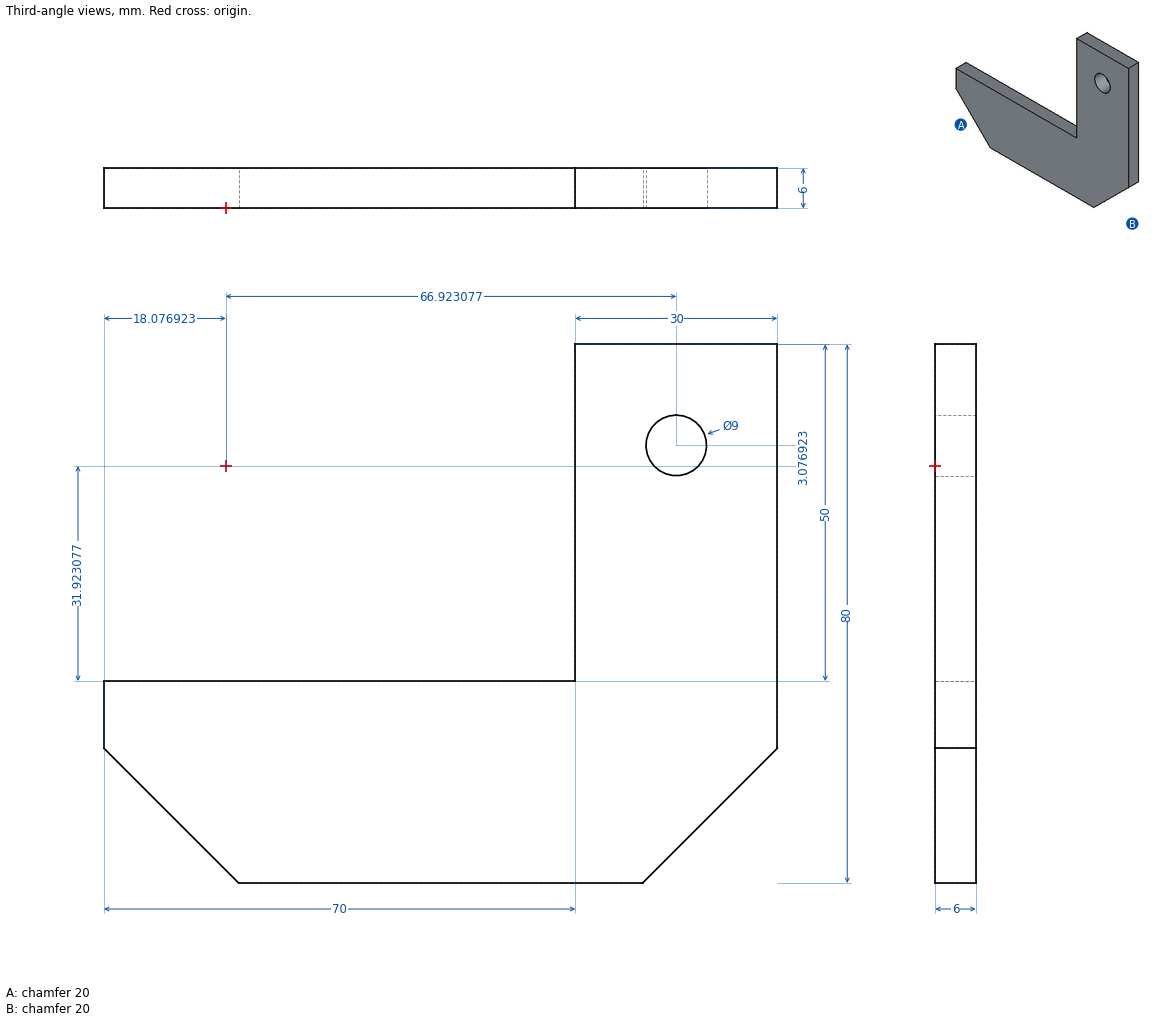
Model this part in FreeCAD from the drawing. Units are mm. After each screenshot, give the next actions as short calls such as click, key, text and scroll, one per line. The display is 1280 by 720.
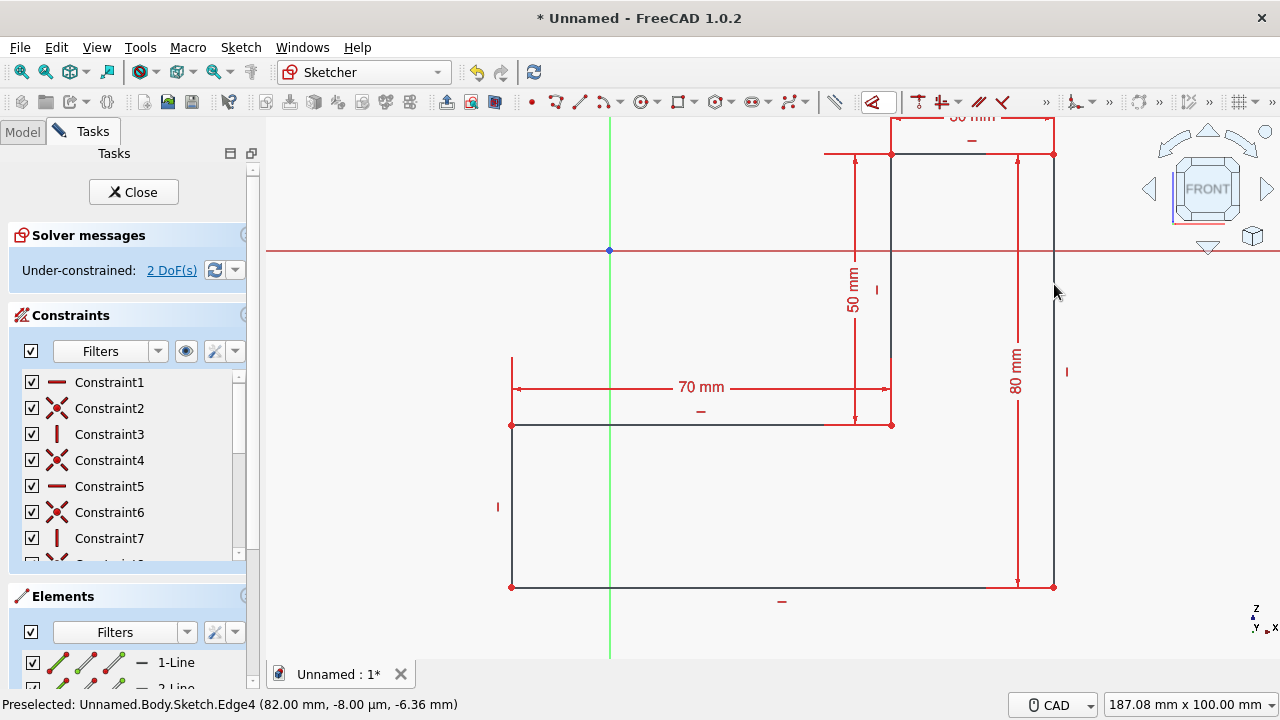
click(512, 425)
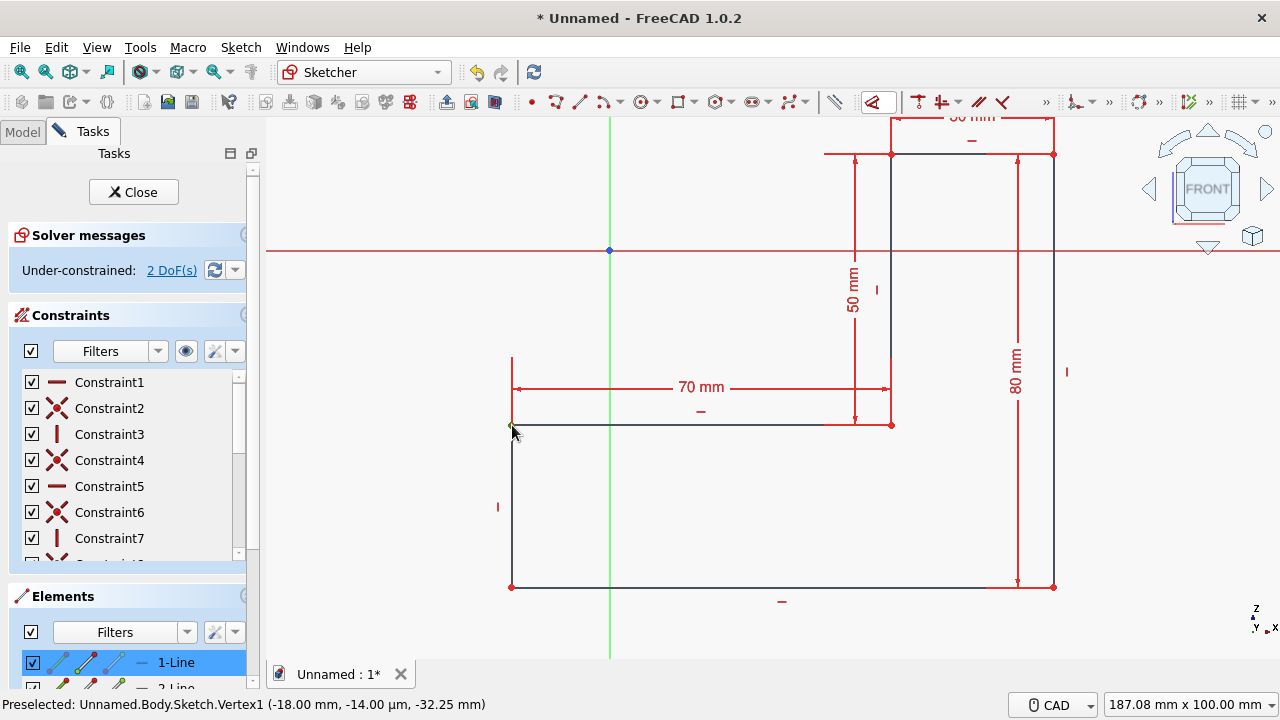
click(890, 102)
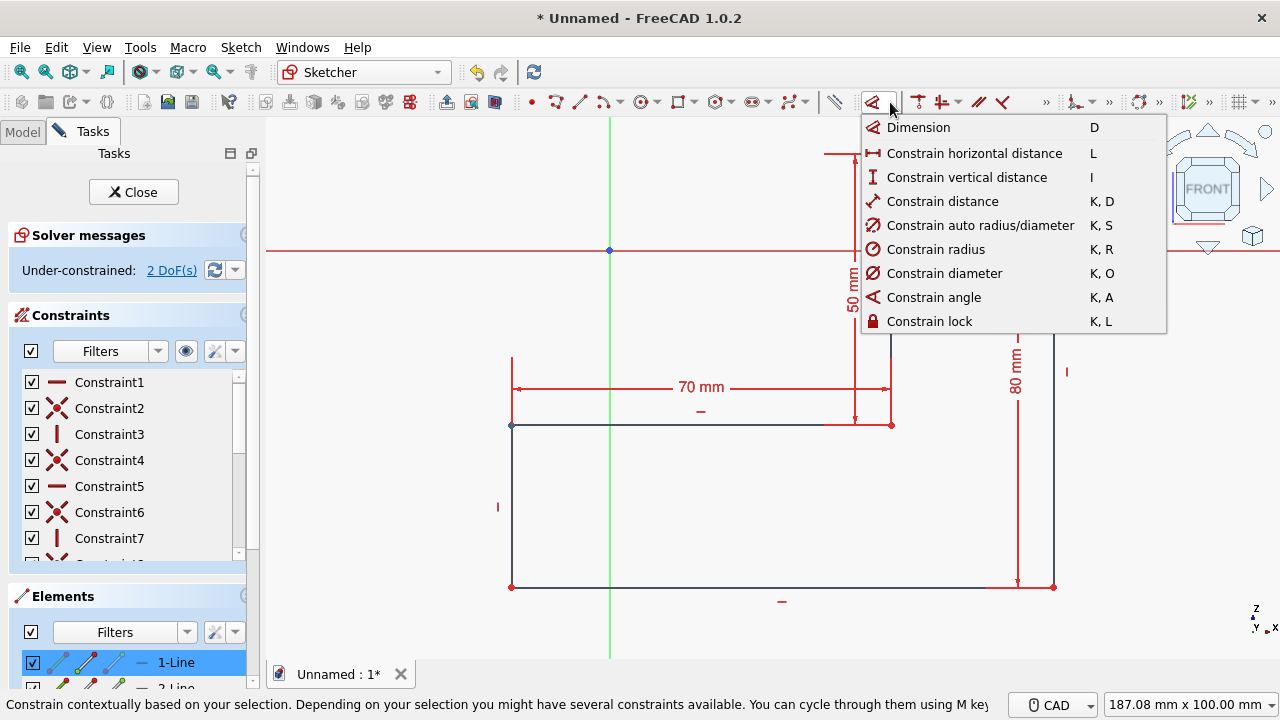
click(1014, 153)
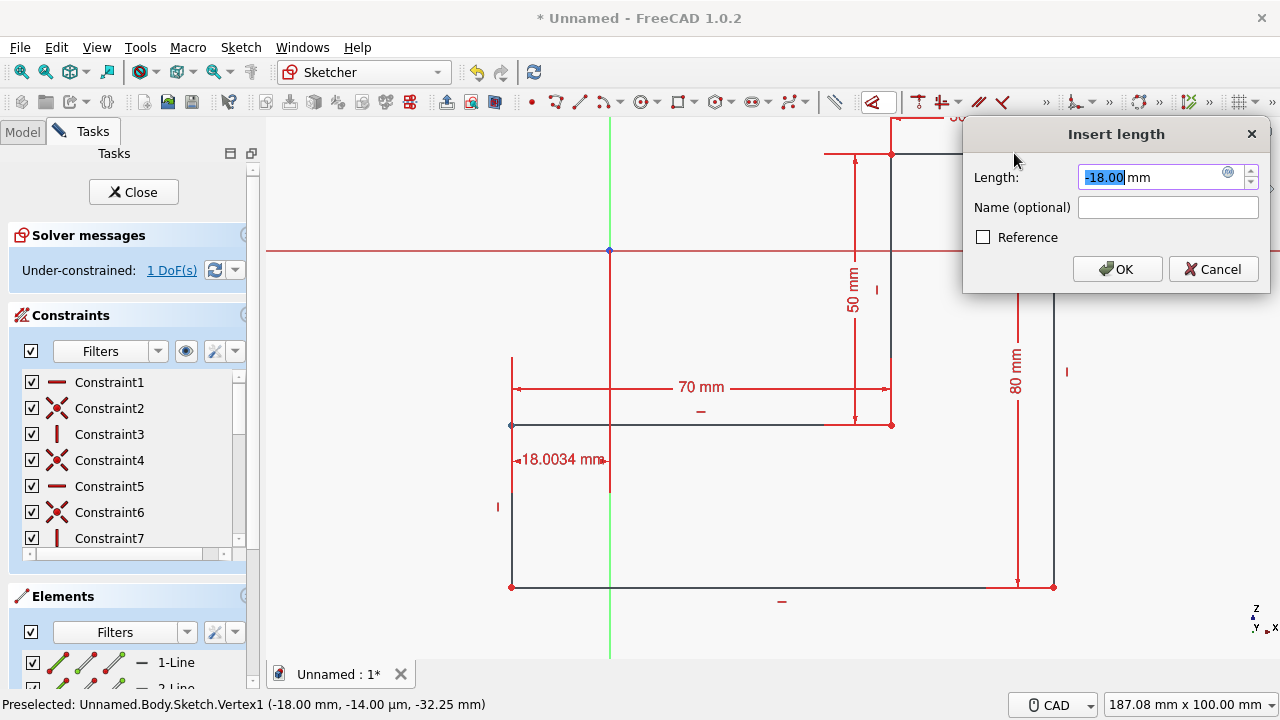
text(-18.076923)
key(Return)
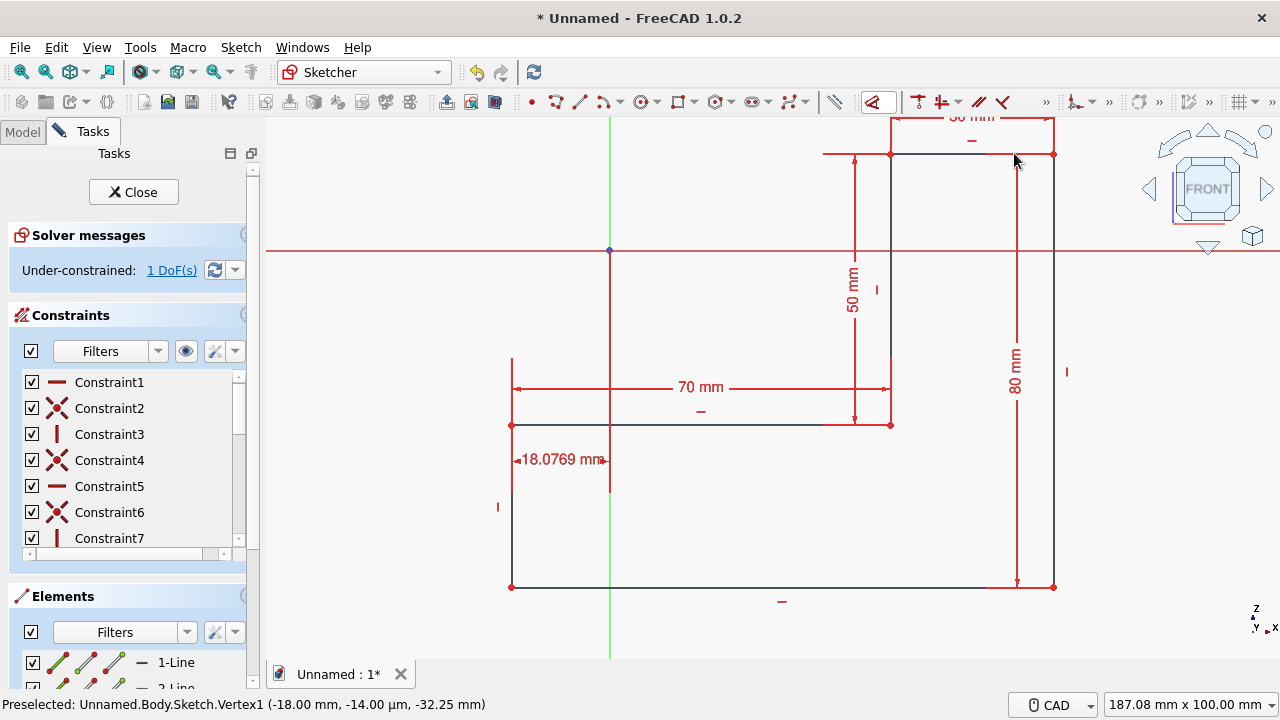
click(512, 425)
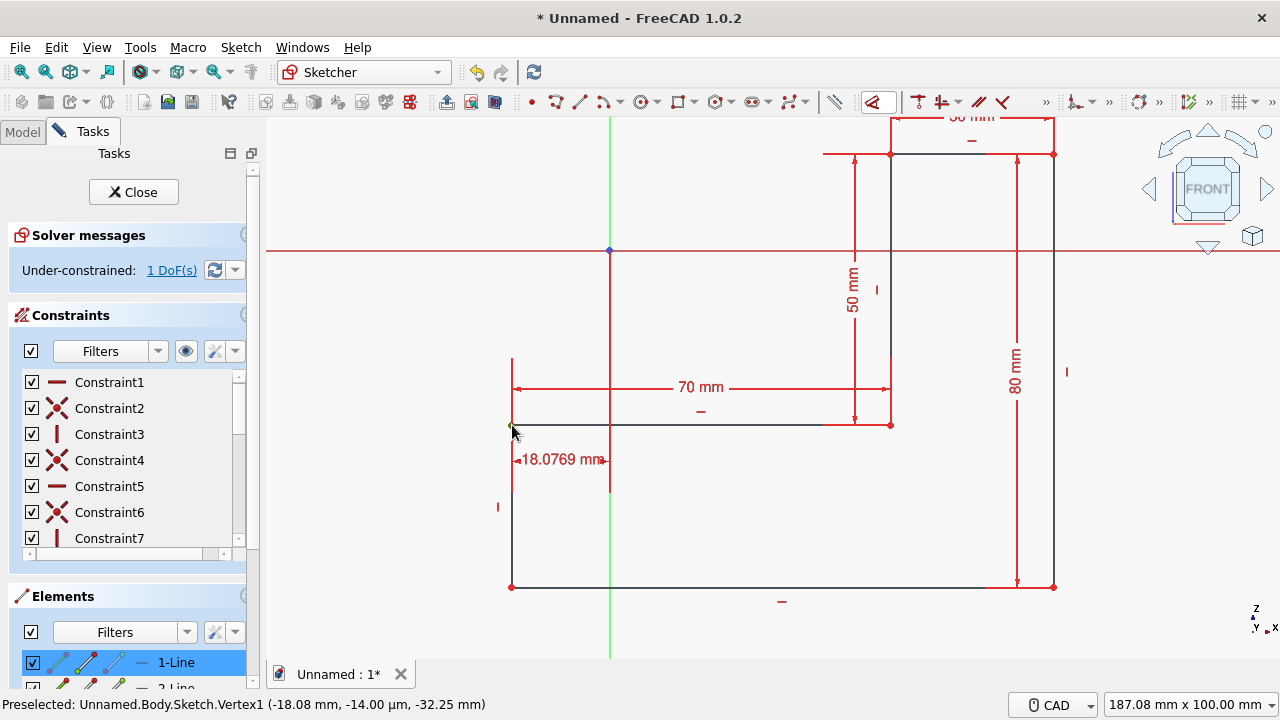
click(890, 102)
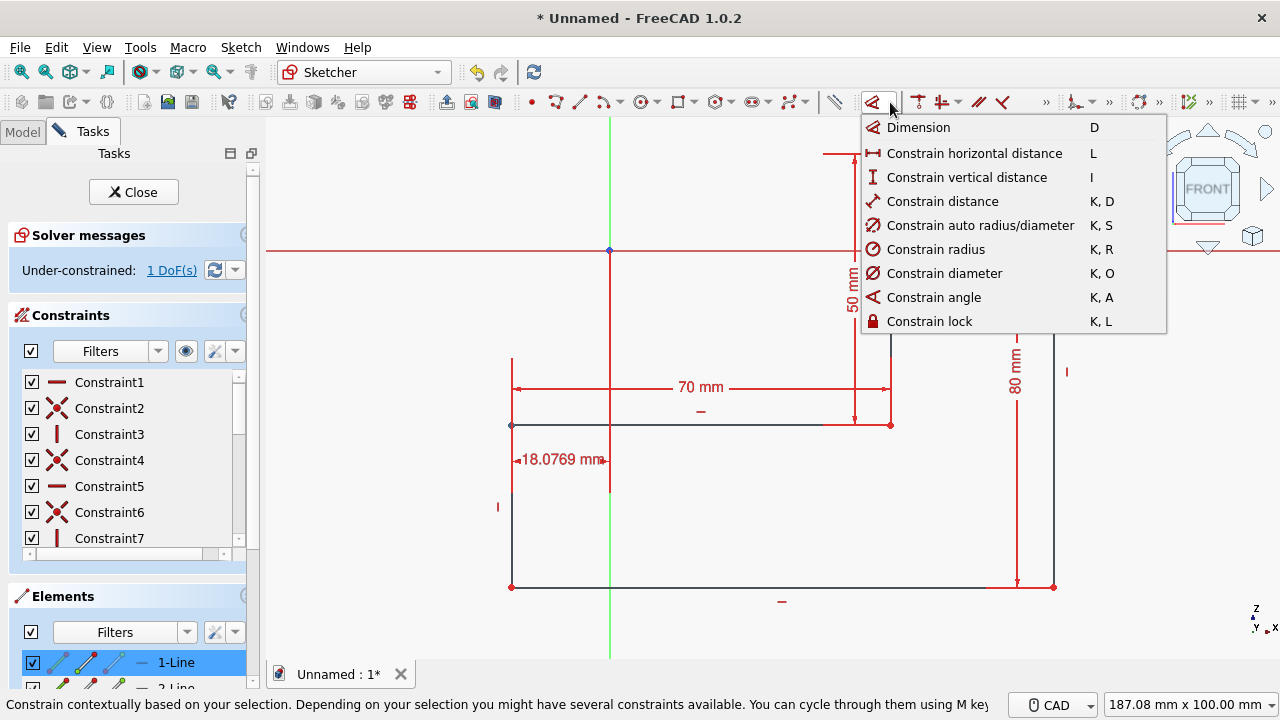
click(1014, 177)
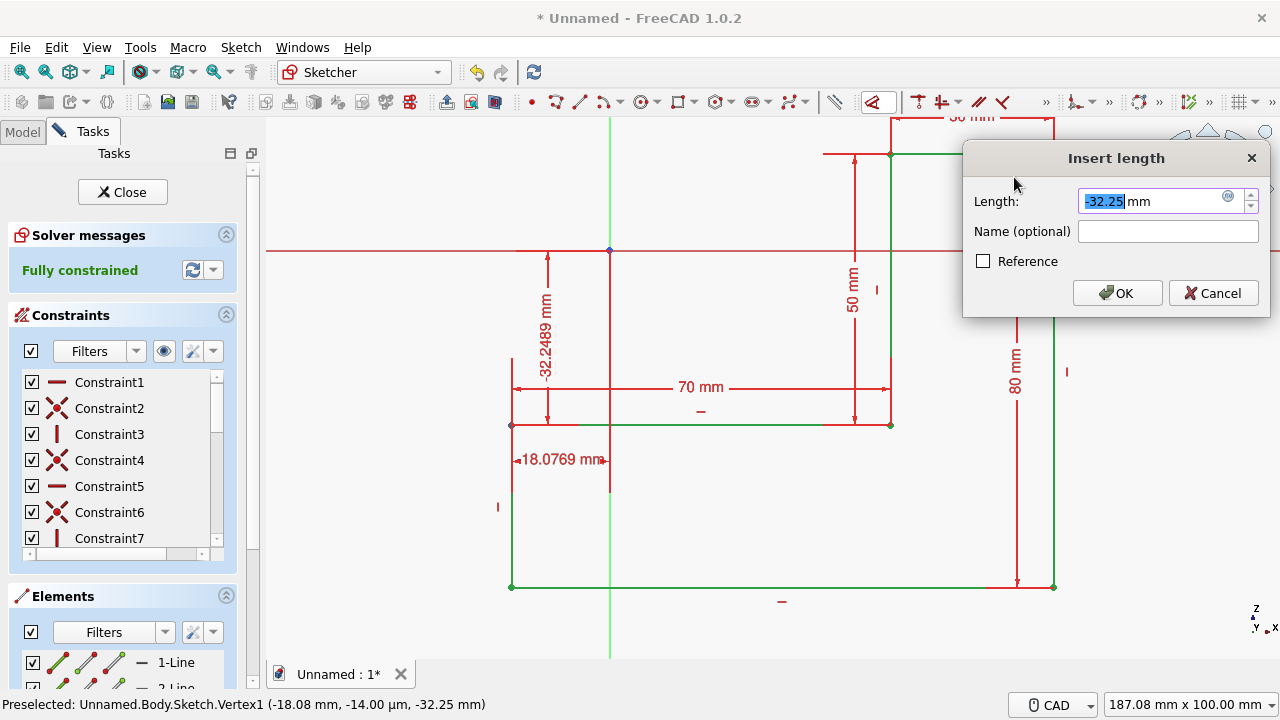
text(-31.923077)
key(Return)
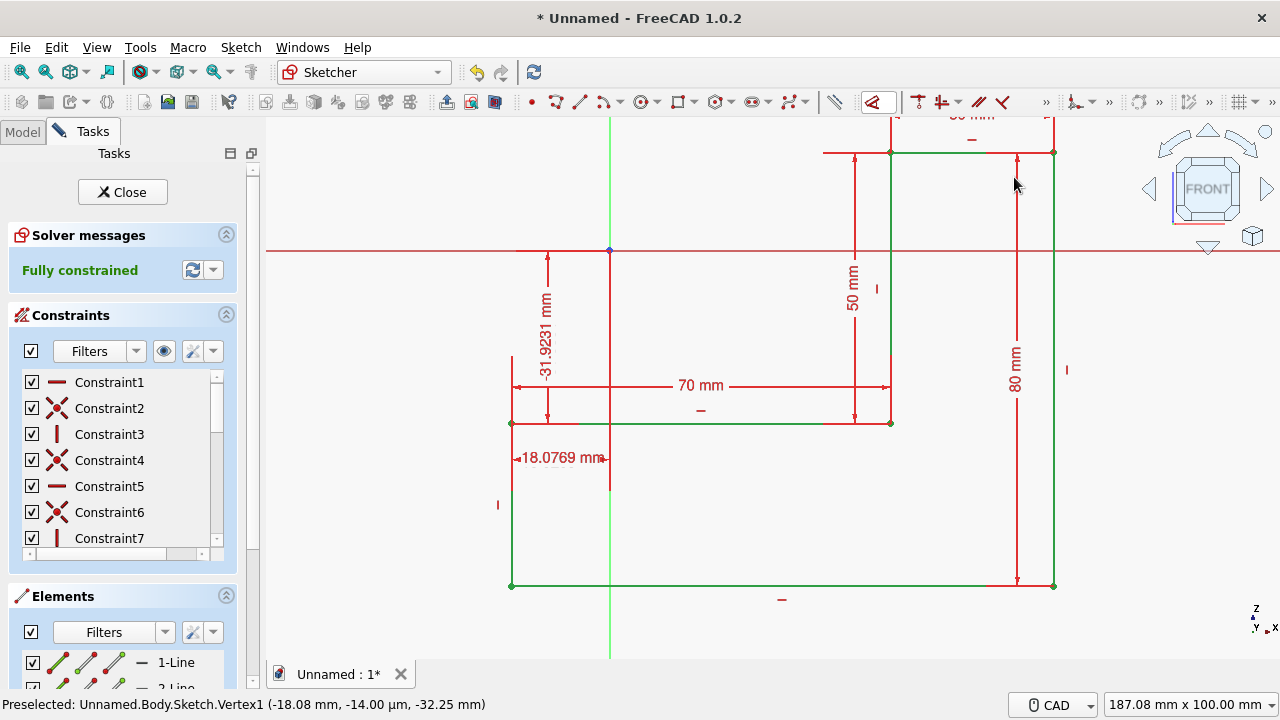
click(123, 192)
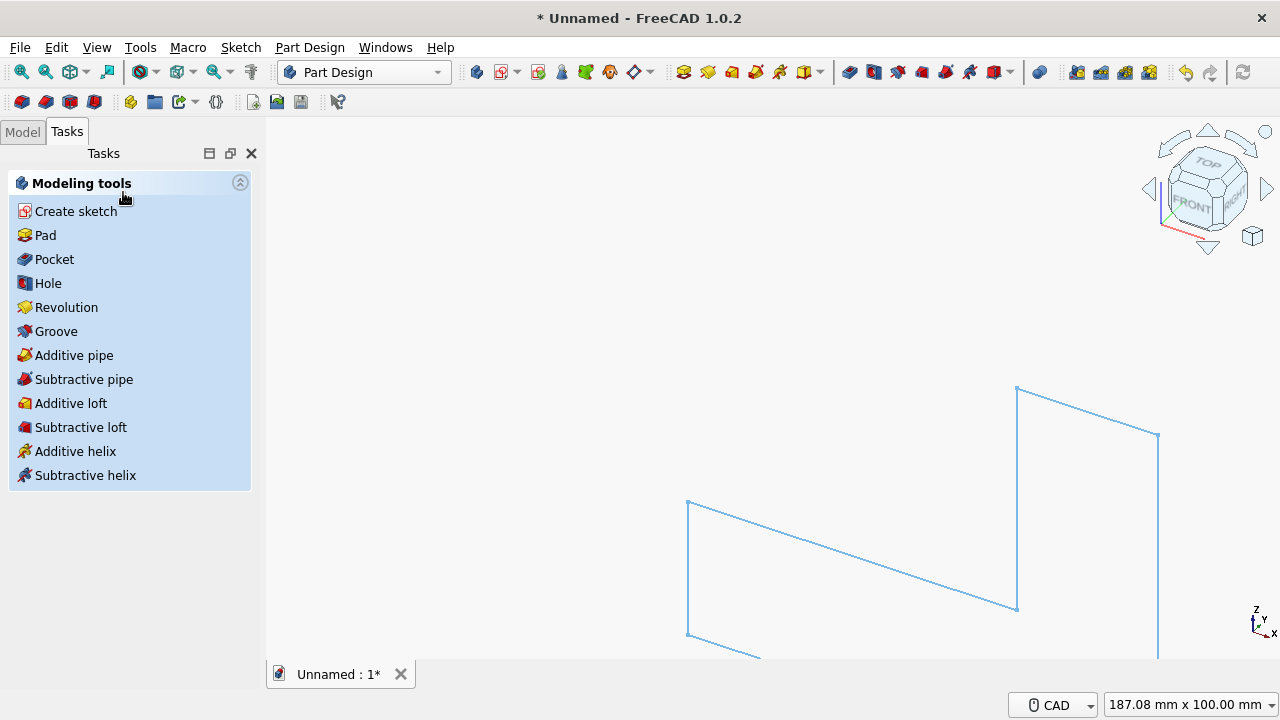
click(684, 72)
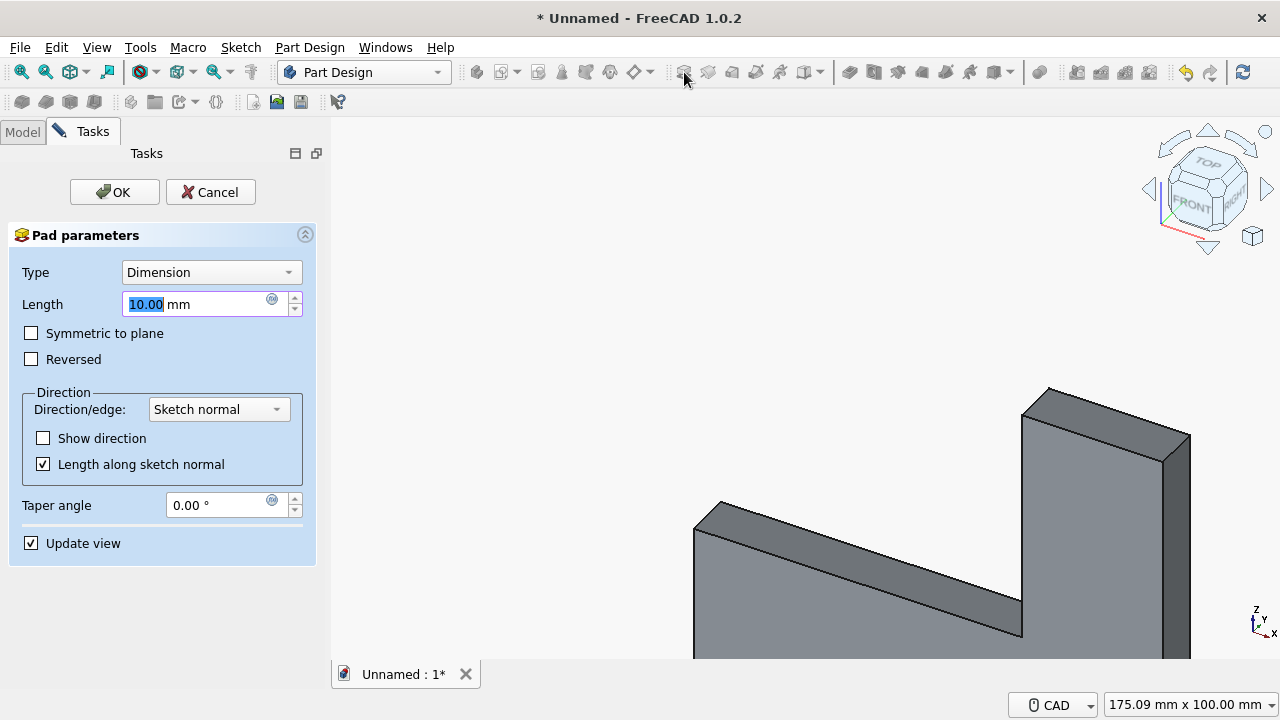
text(6)
key(Tab)